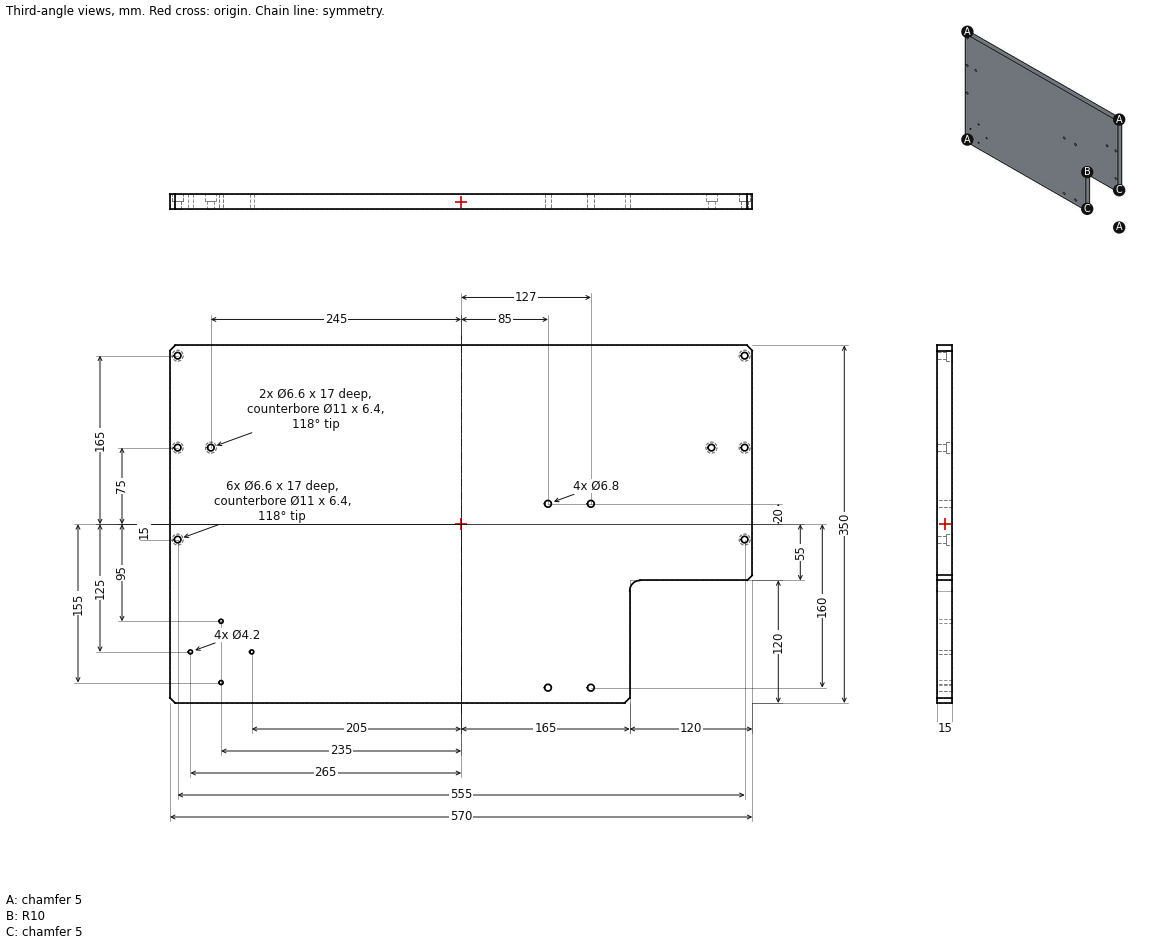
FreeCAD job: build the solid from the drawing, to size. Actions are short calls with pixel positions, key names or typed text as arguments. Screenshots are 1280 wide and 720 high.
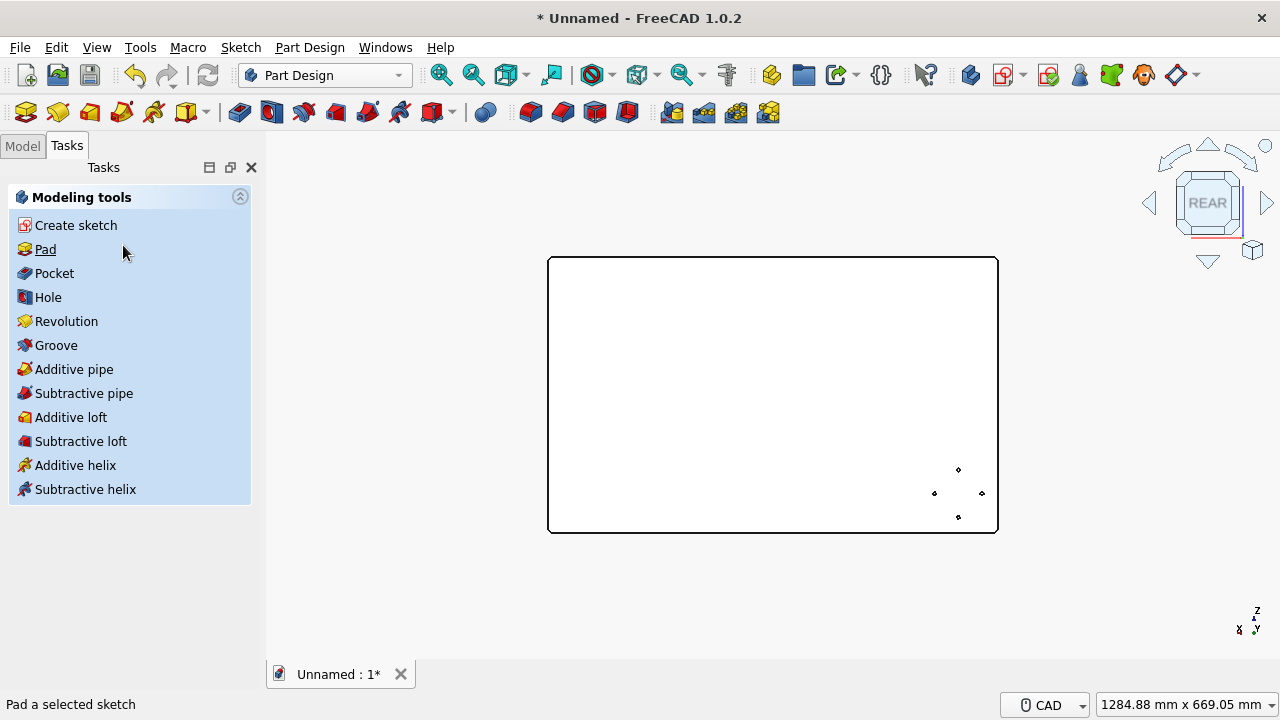
click(240, 112)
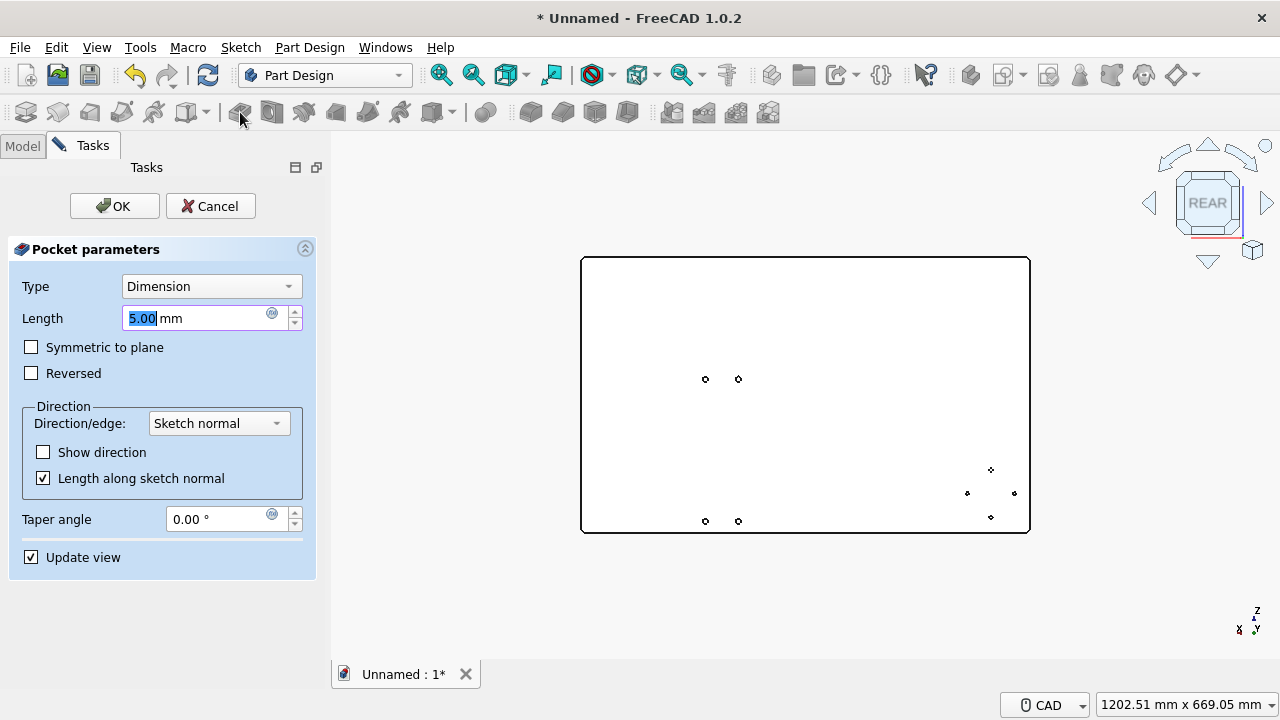
click(212, 286)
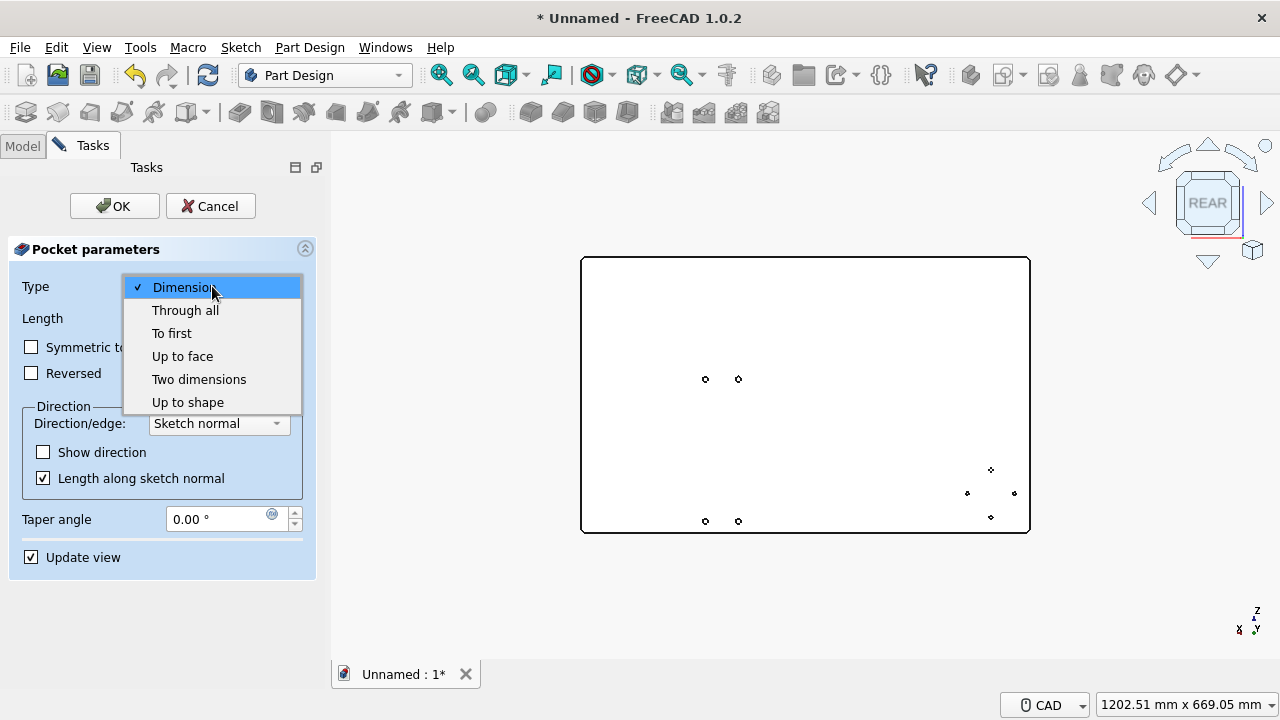
click(212, 310)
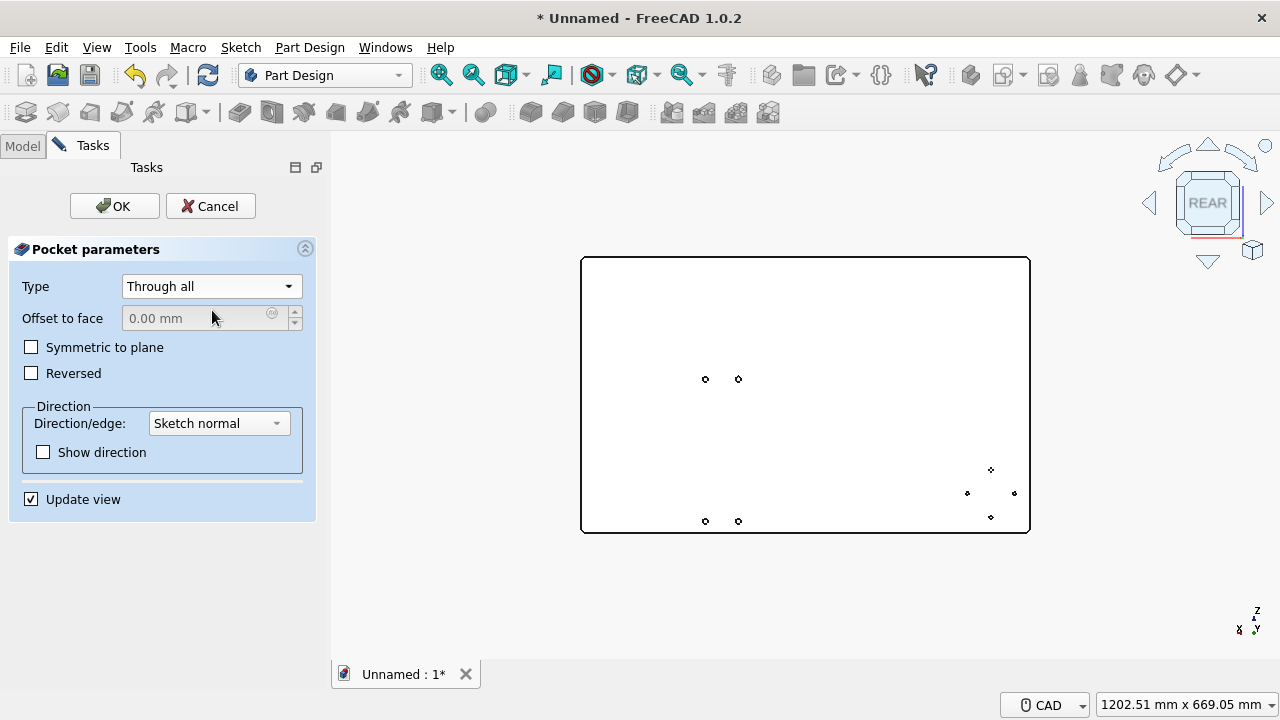
click(115, 206)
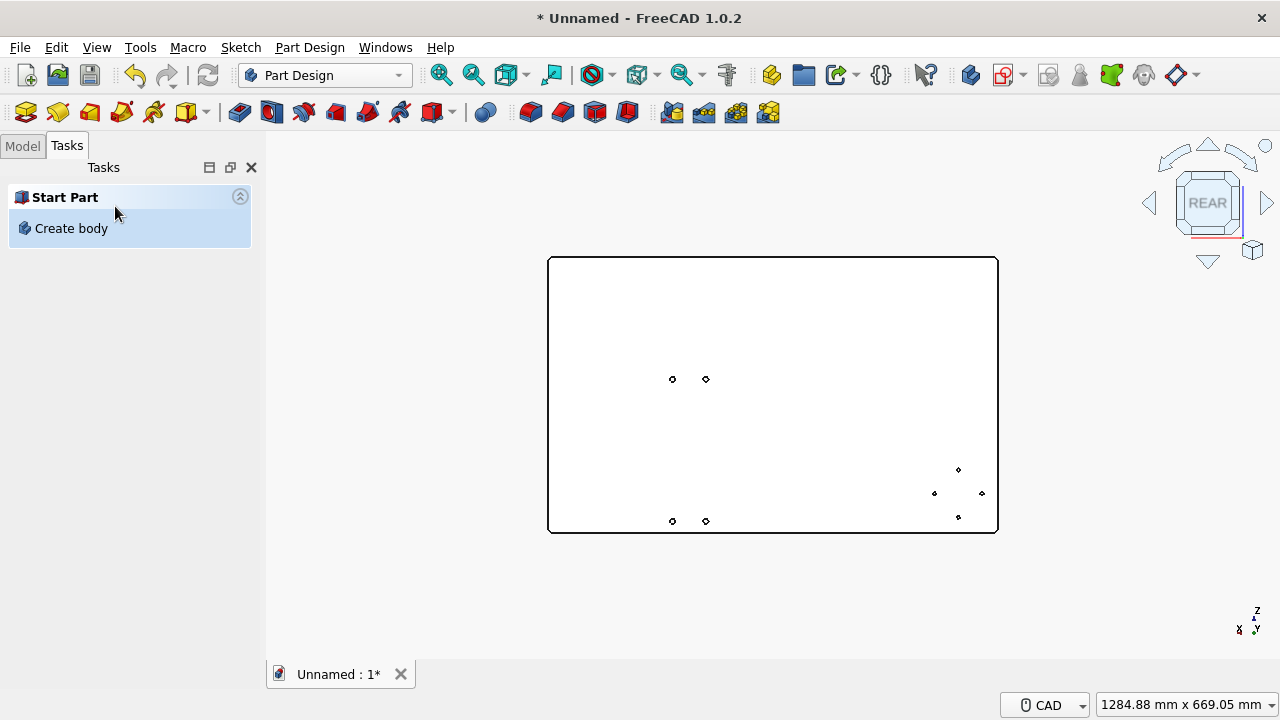
click(837, 394)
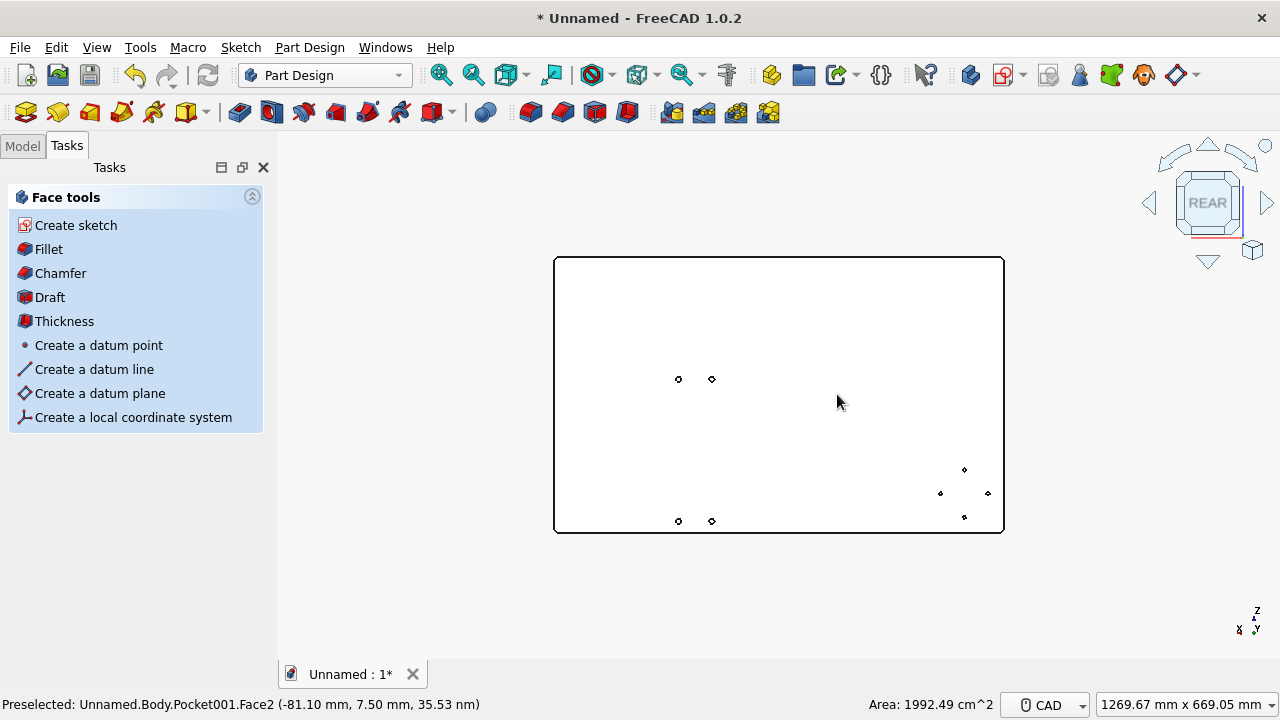
click(1004, 76)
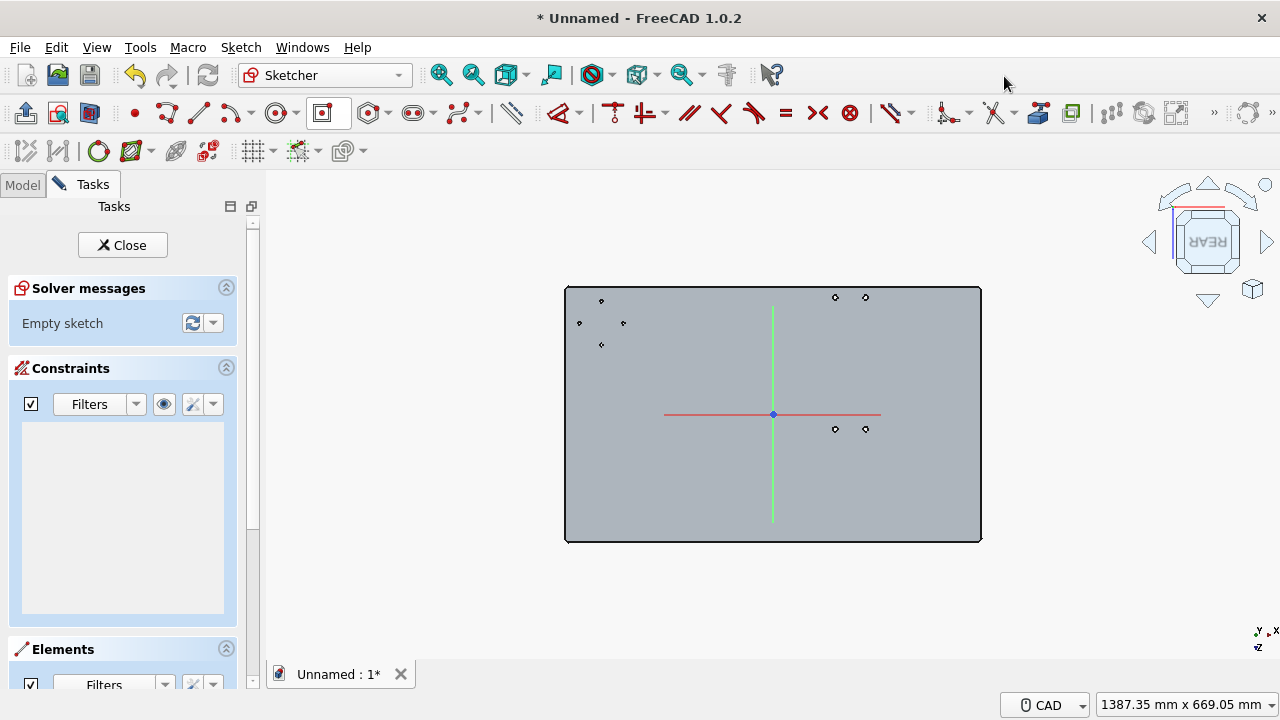
scroll(912, 581, up, 2)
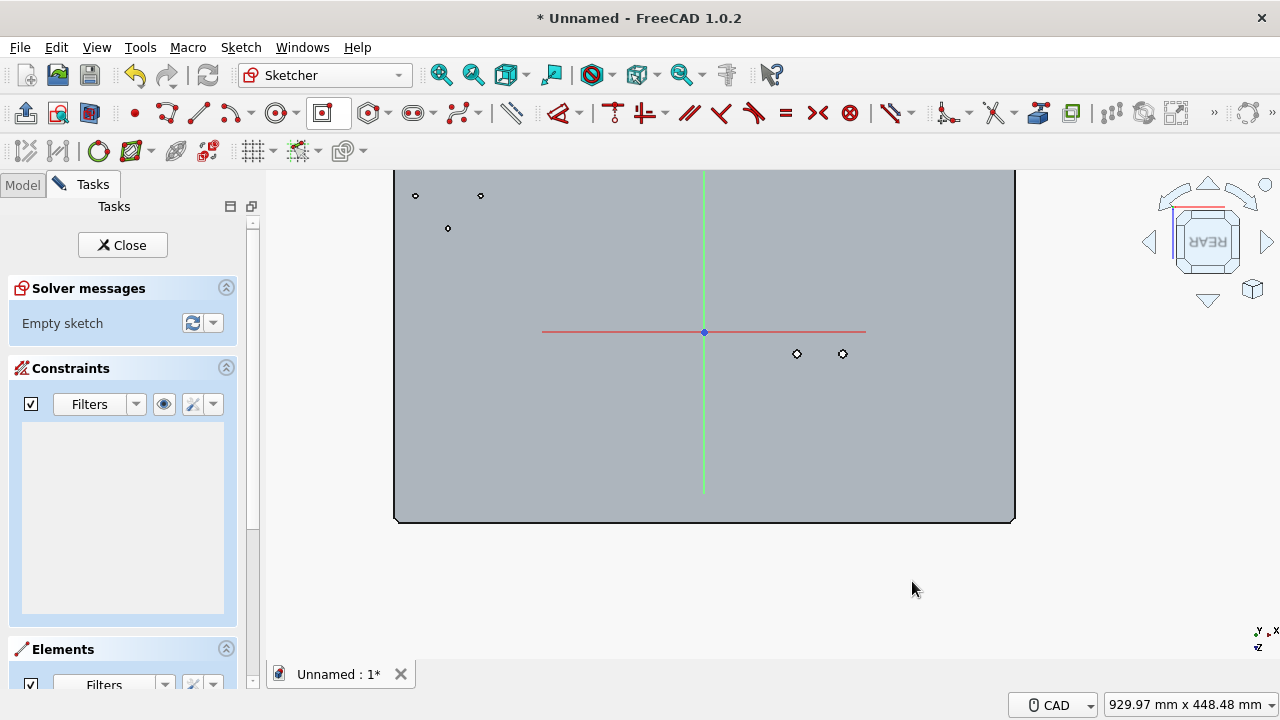
click(276, 114)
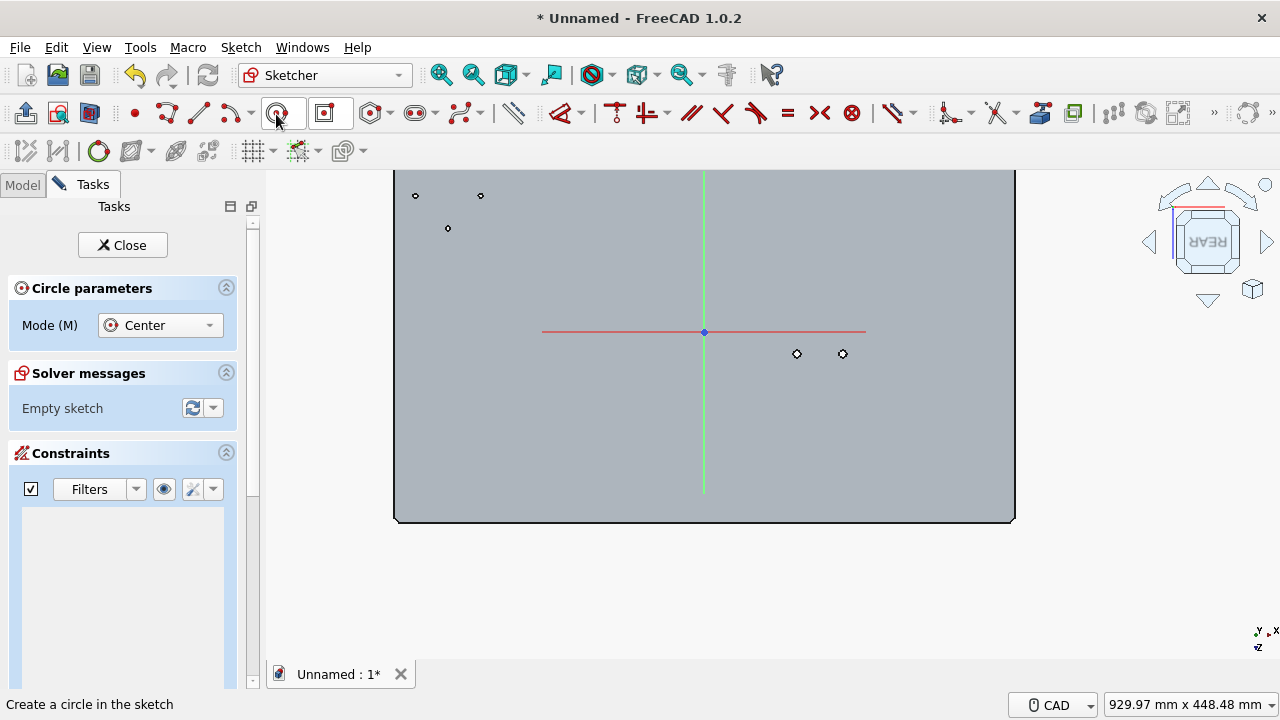
scroll(402, 316, up, 10)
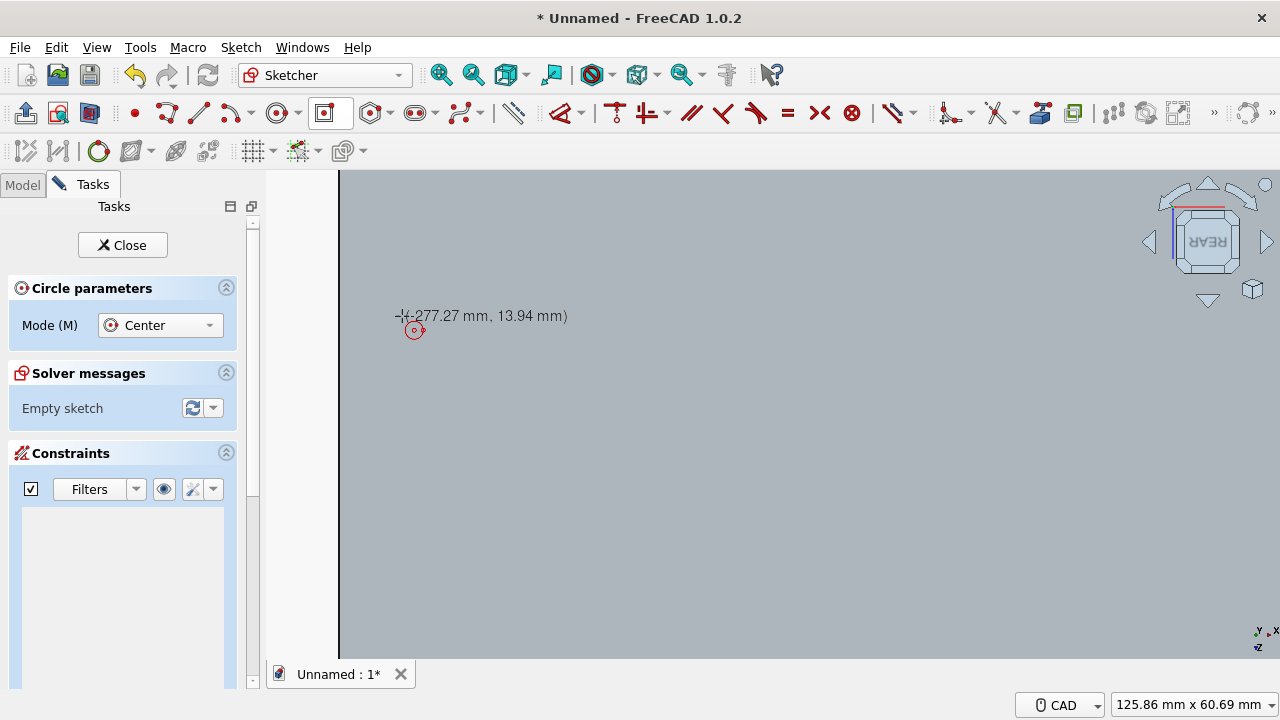
scroll(402, 317, down, 10)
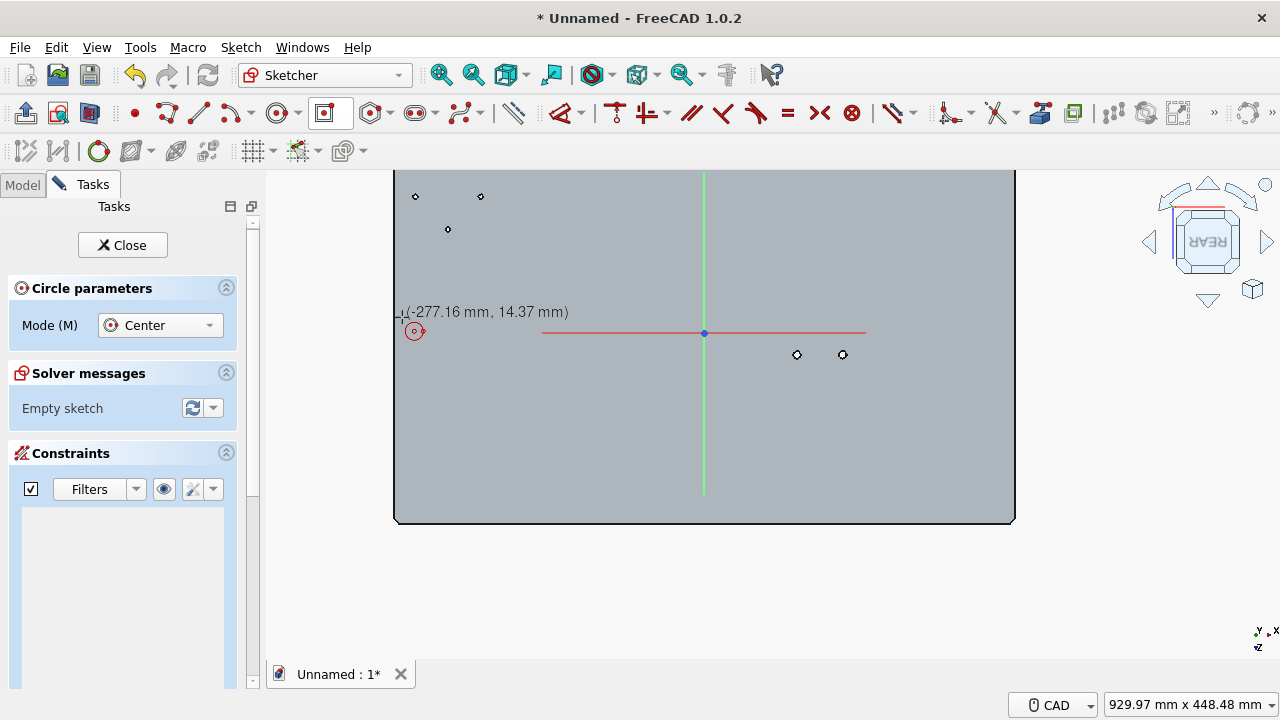
click(402, 317)
move(404, 314)